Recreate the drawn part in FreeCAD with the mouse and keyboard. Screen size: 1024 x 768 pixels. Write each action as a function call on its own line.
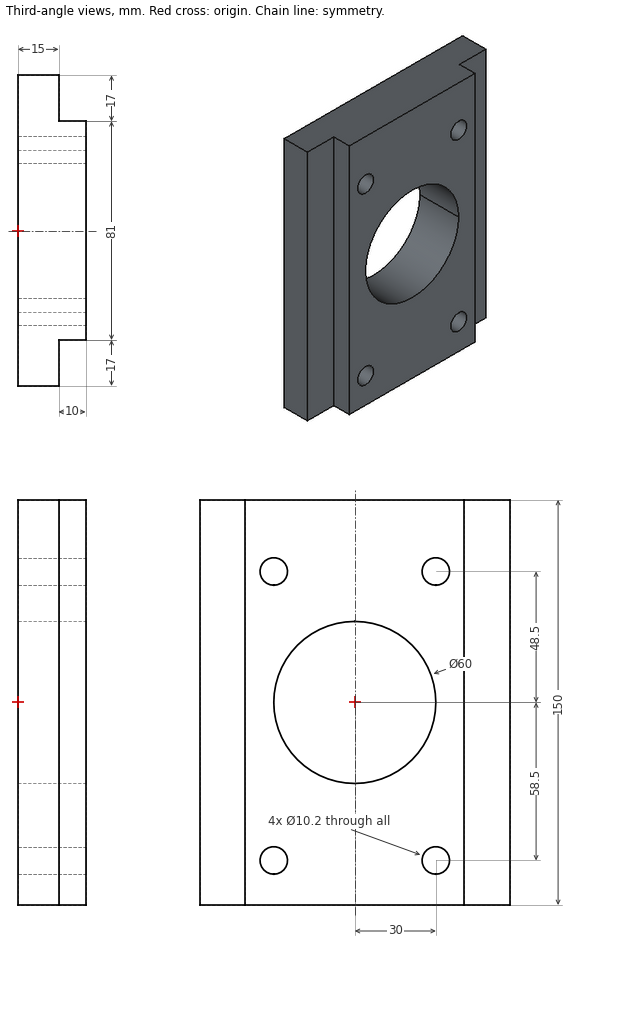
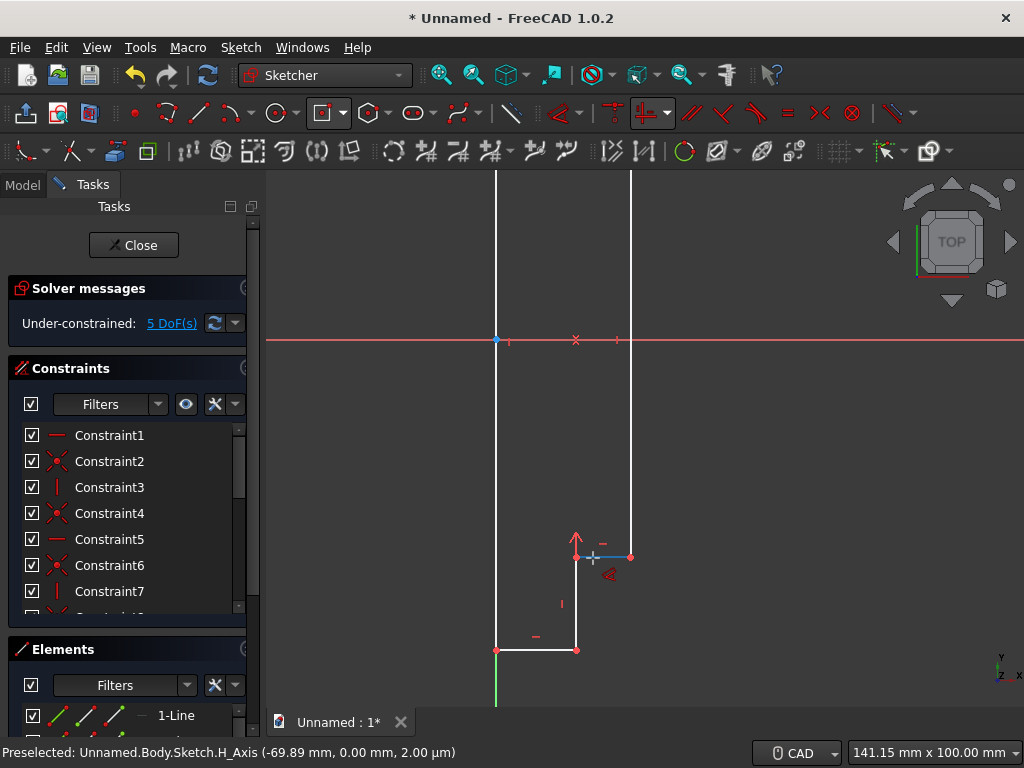
click(593, 557)
click(604, 591)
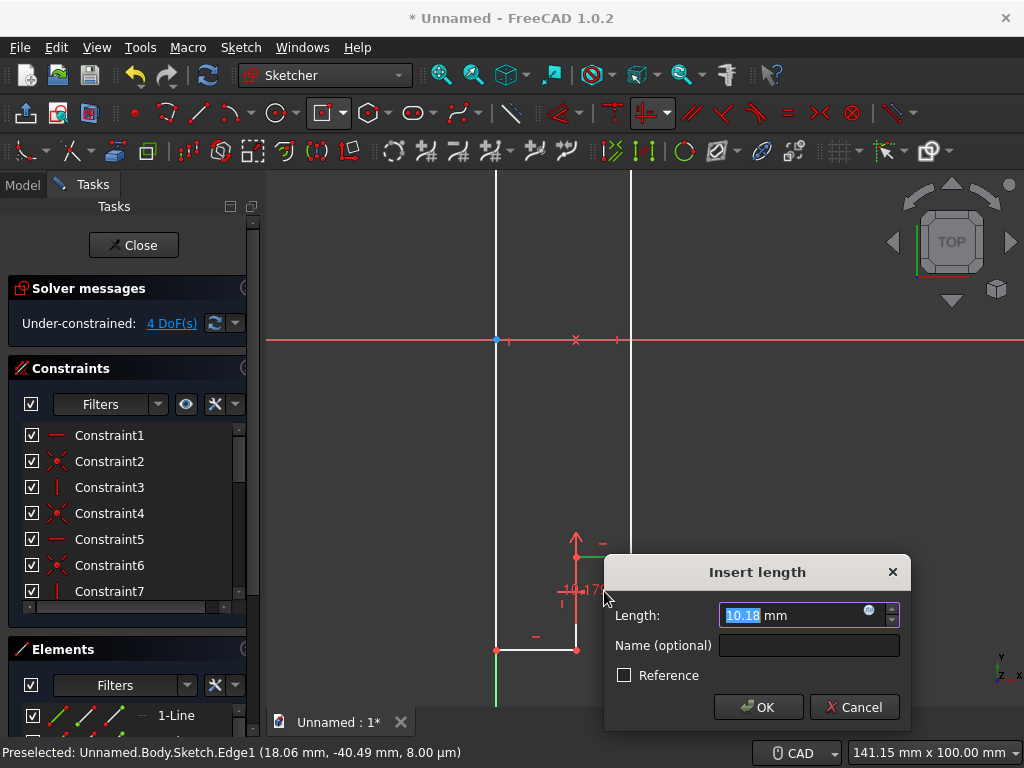
text(10)
key(Return)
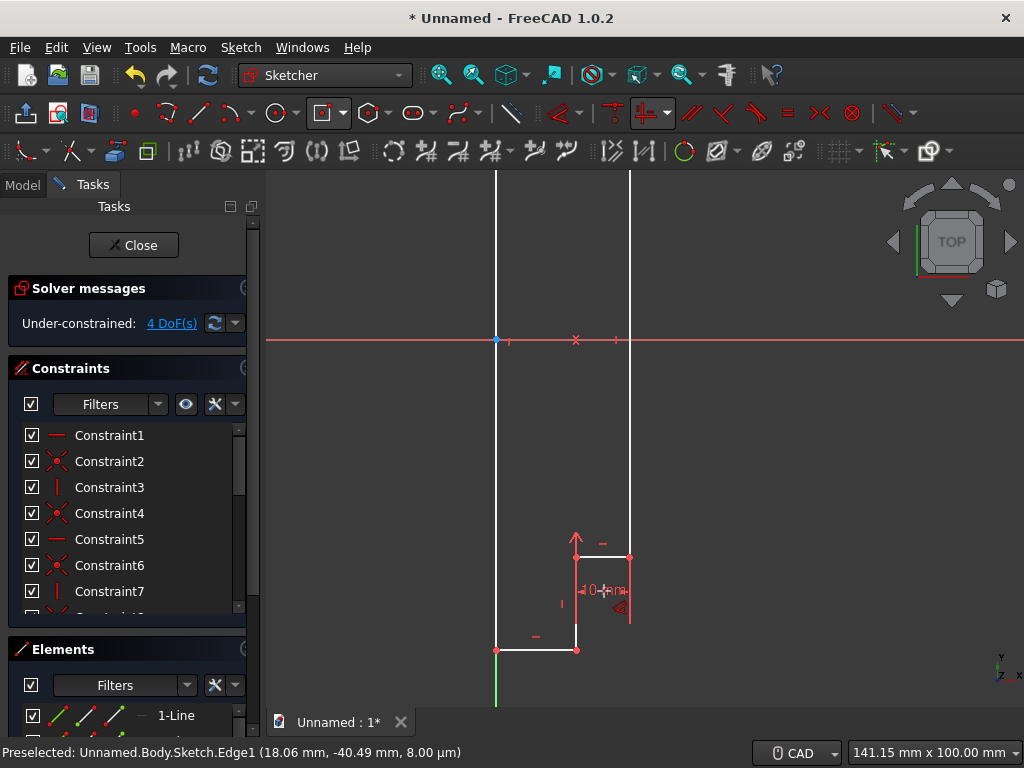
click(630, 427)
click(664, 378)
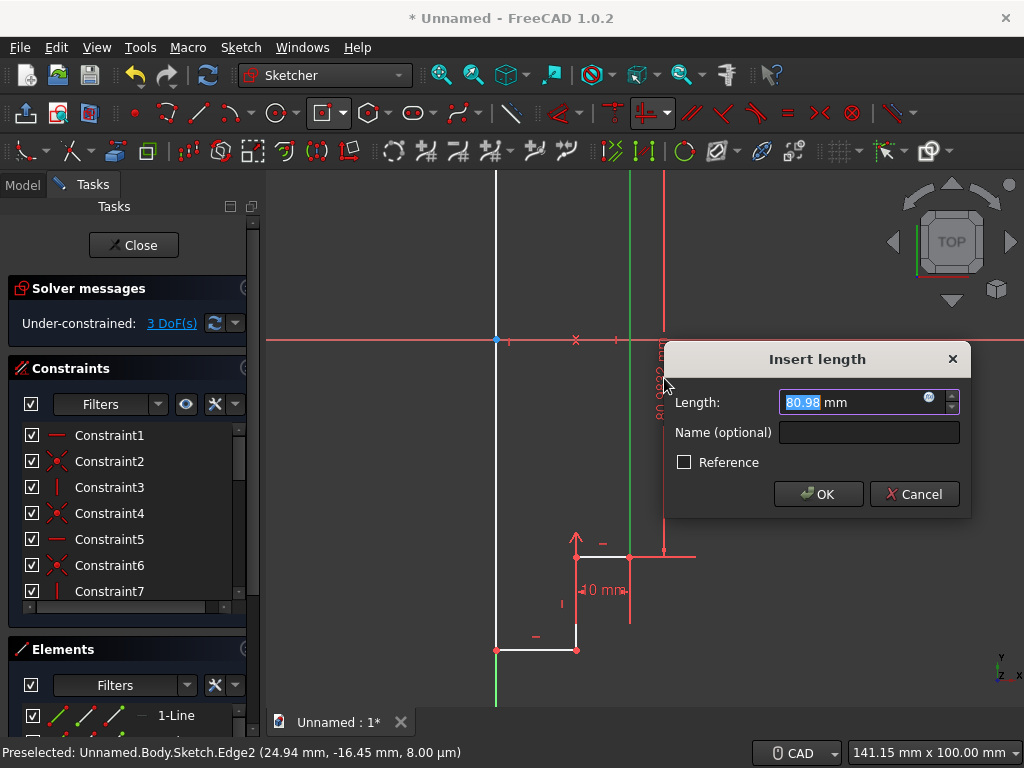
text(81)
key(Return)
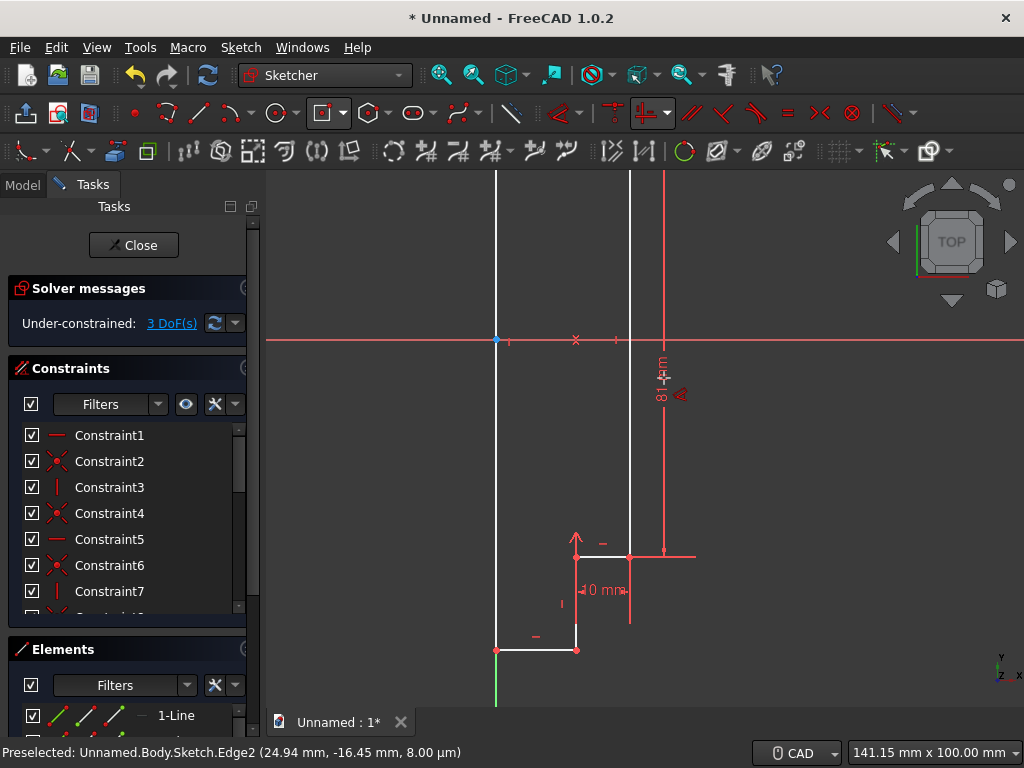
scroll(593, 559, down, 3)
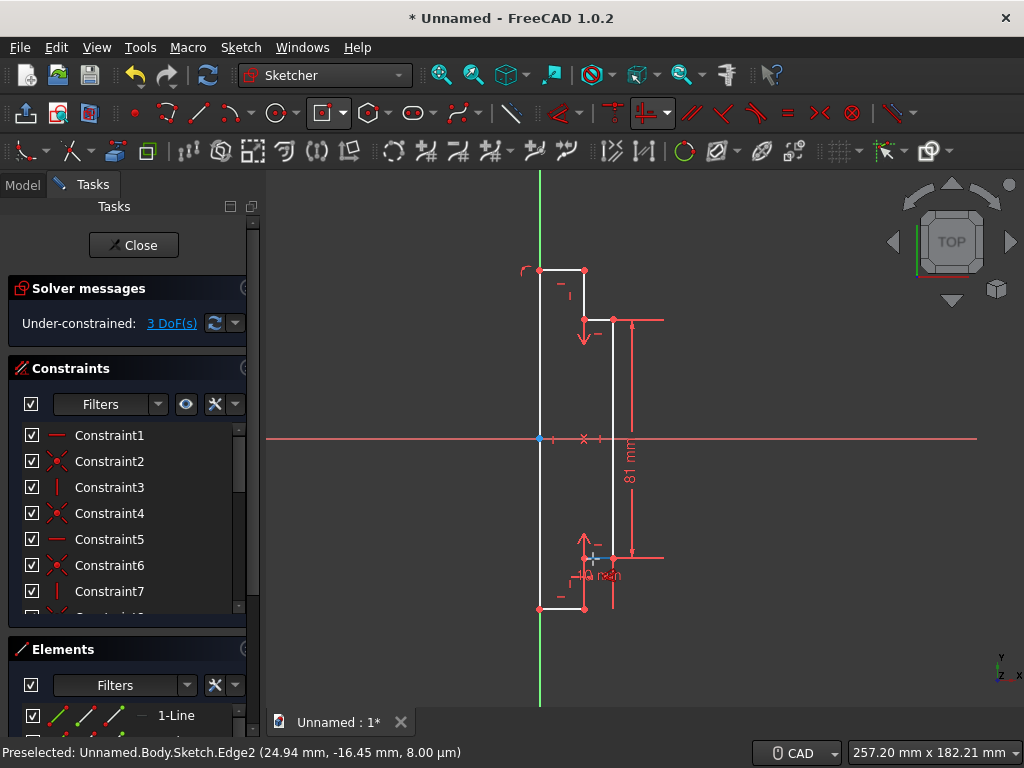
click(584, 305)
click(618, 295)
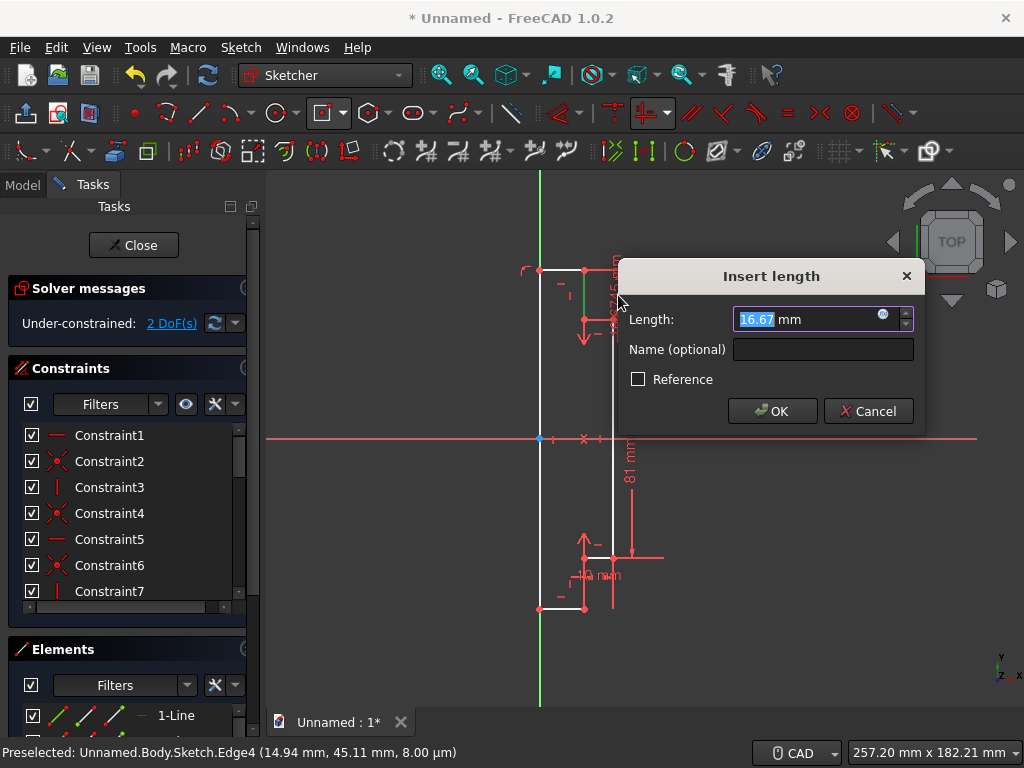
text(17)
key(Return)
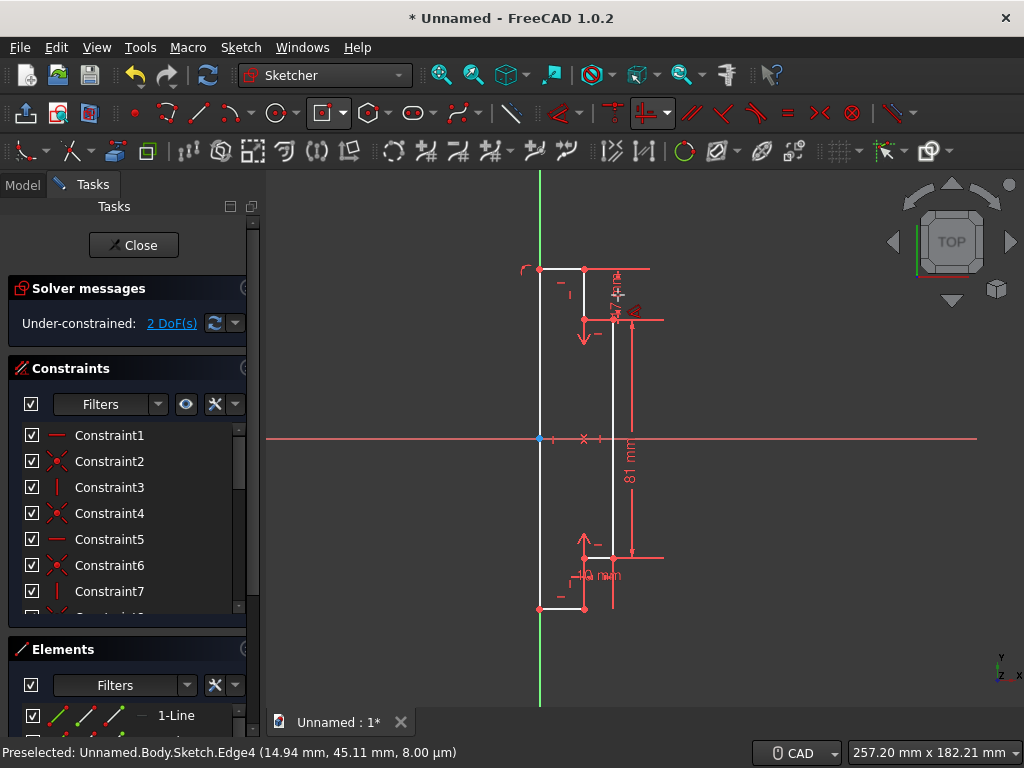
click(571, 269)
click(562, 235)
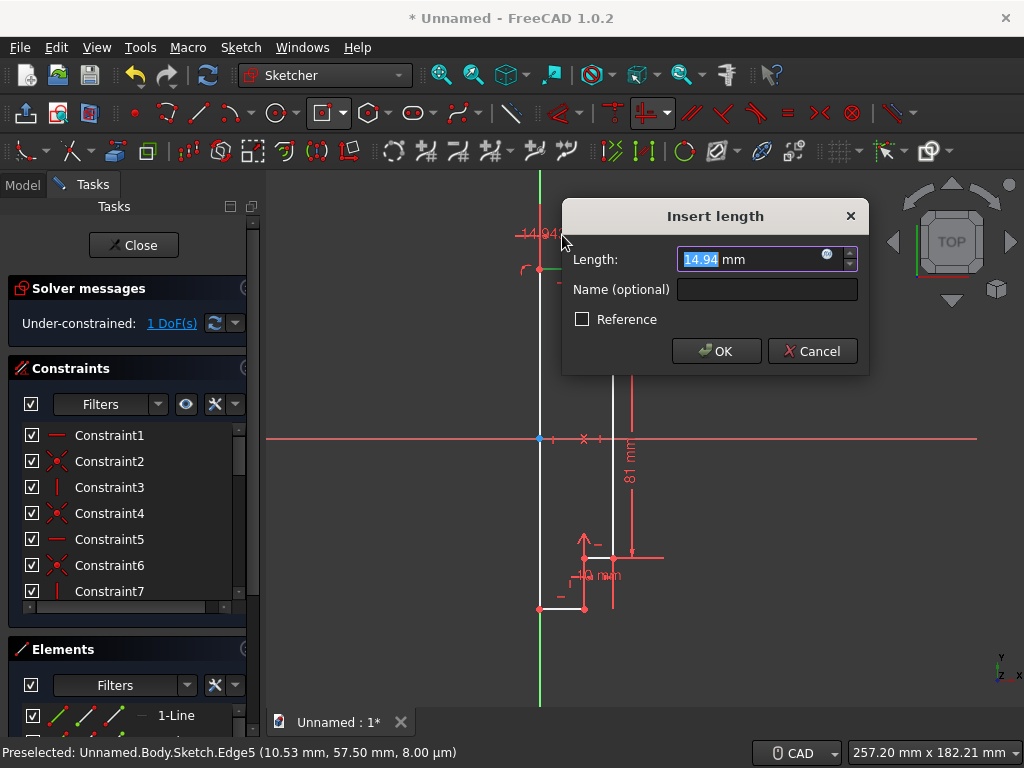
text(15)
key(Return)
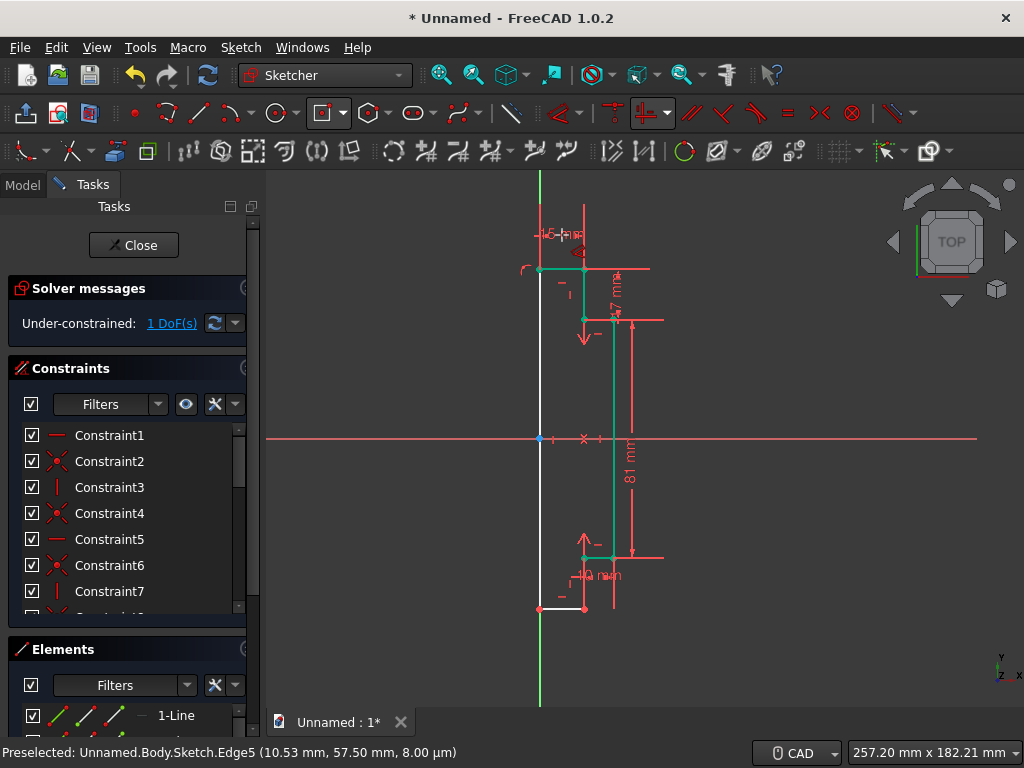
click(584, 594)
click(618, 602)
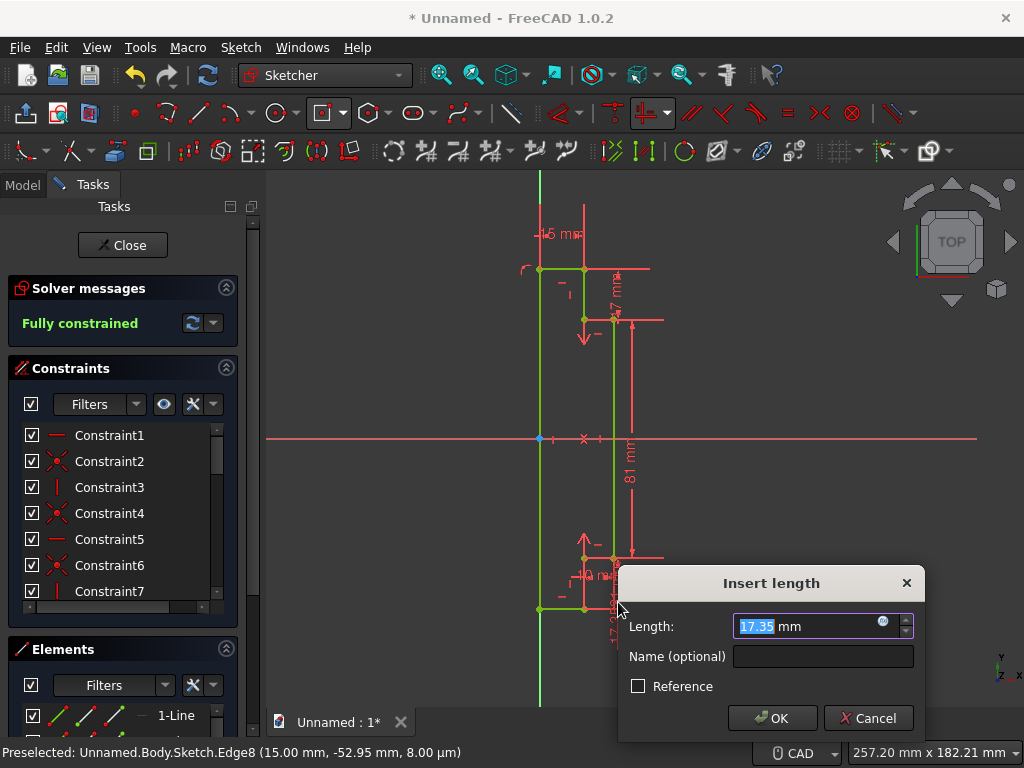
text(17)
key(Return)
key(Escape)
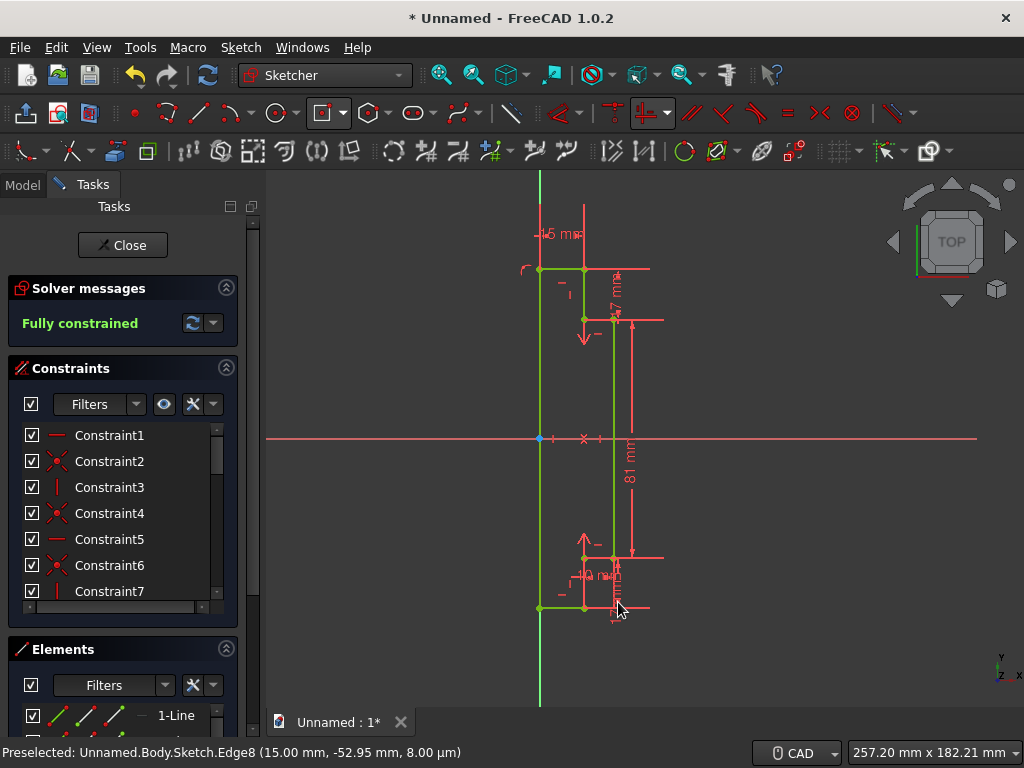
click(123, 245)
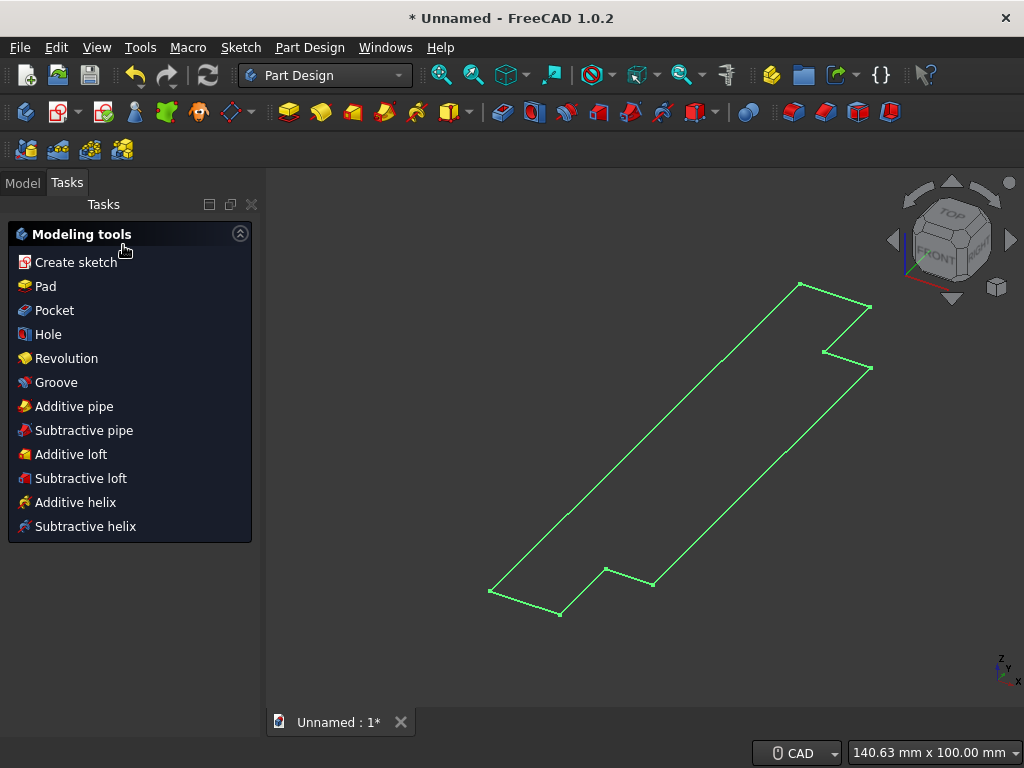
click(290, 112)